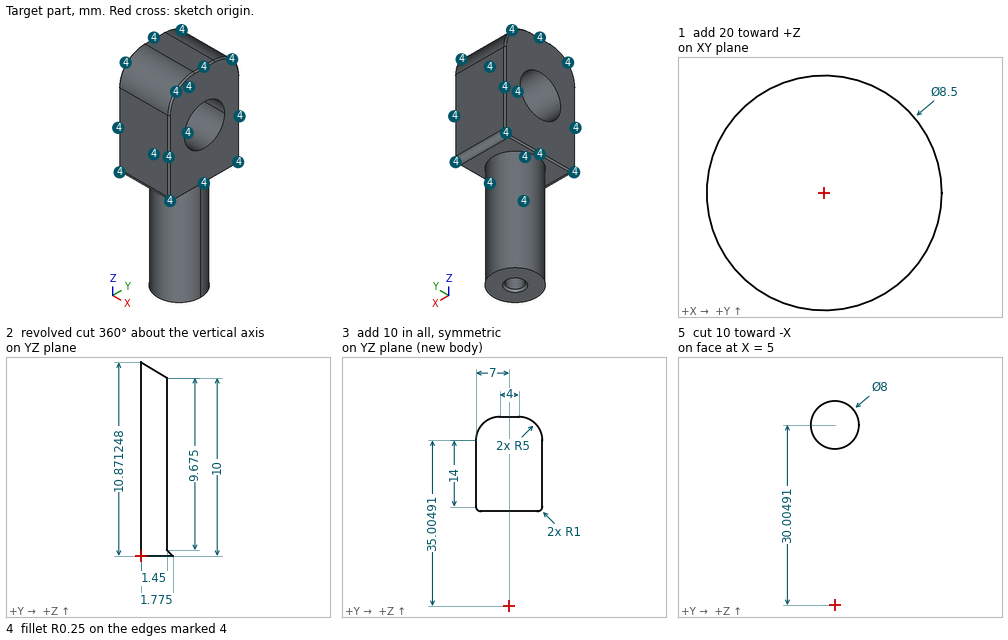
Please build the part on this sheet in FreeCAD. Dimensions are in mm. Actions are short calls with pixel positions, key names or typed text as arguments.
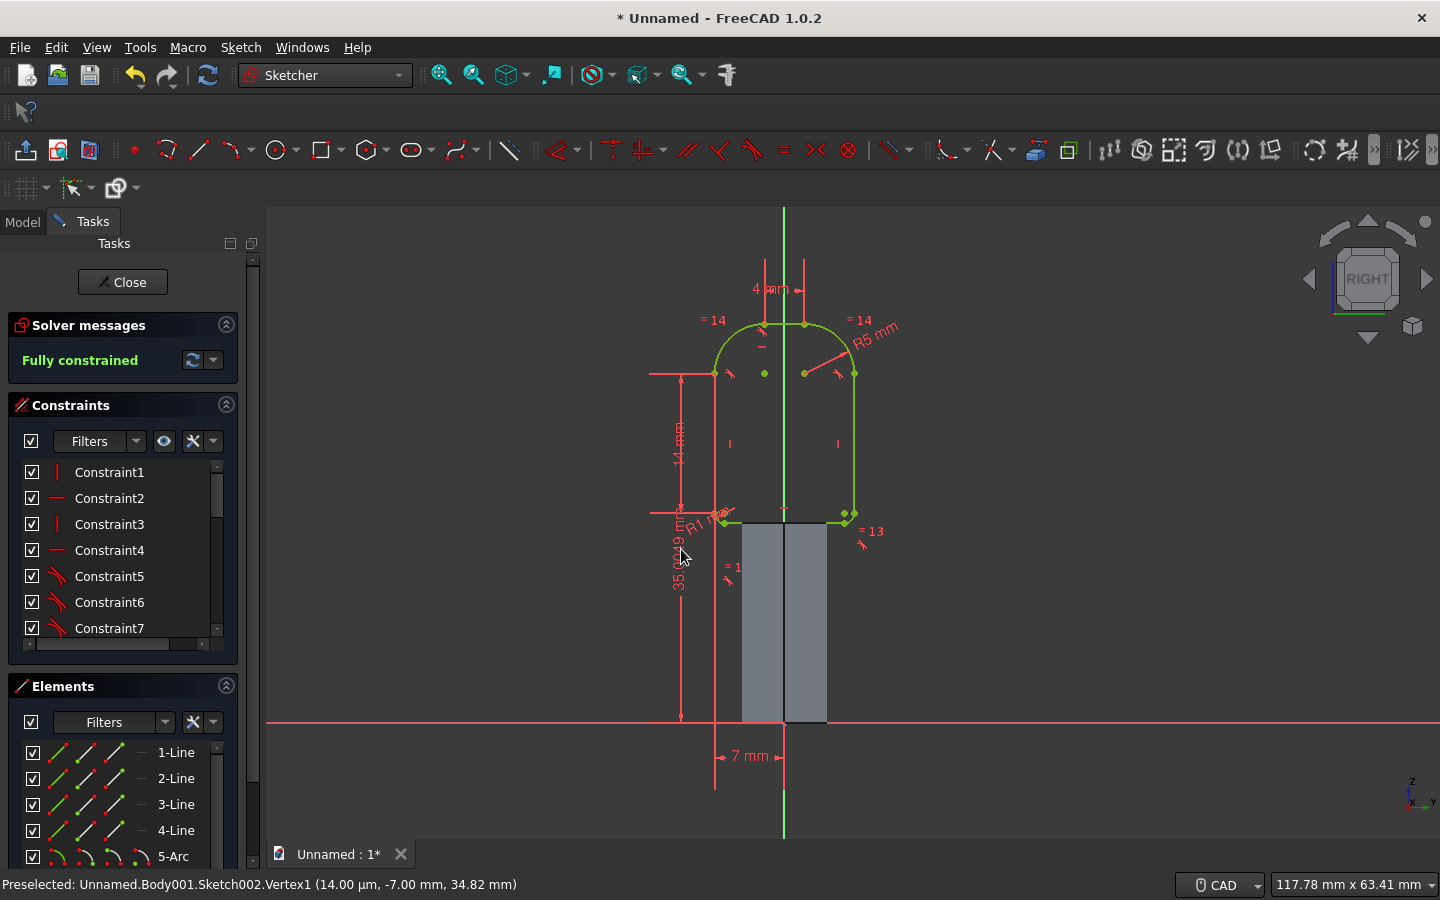
click(123, 282)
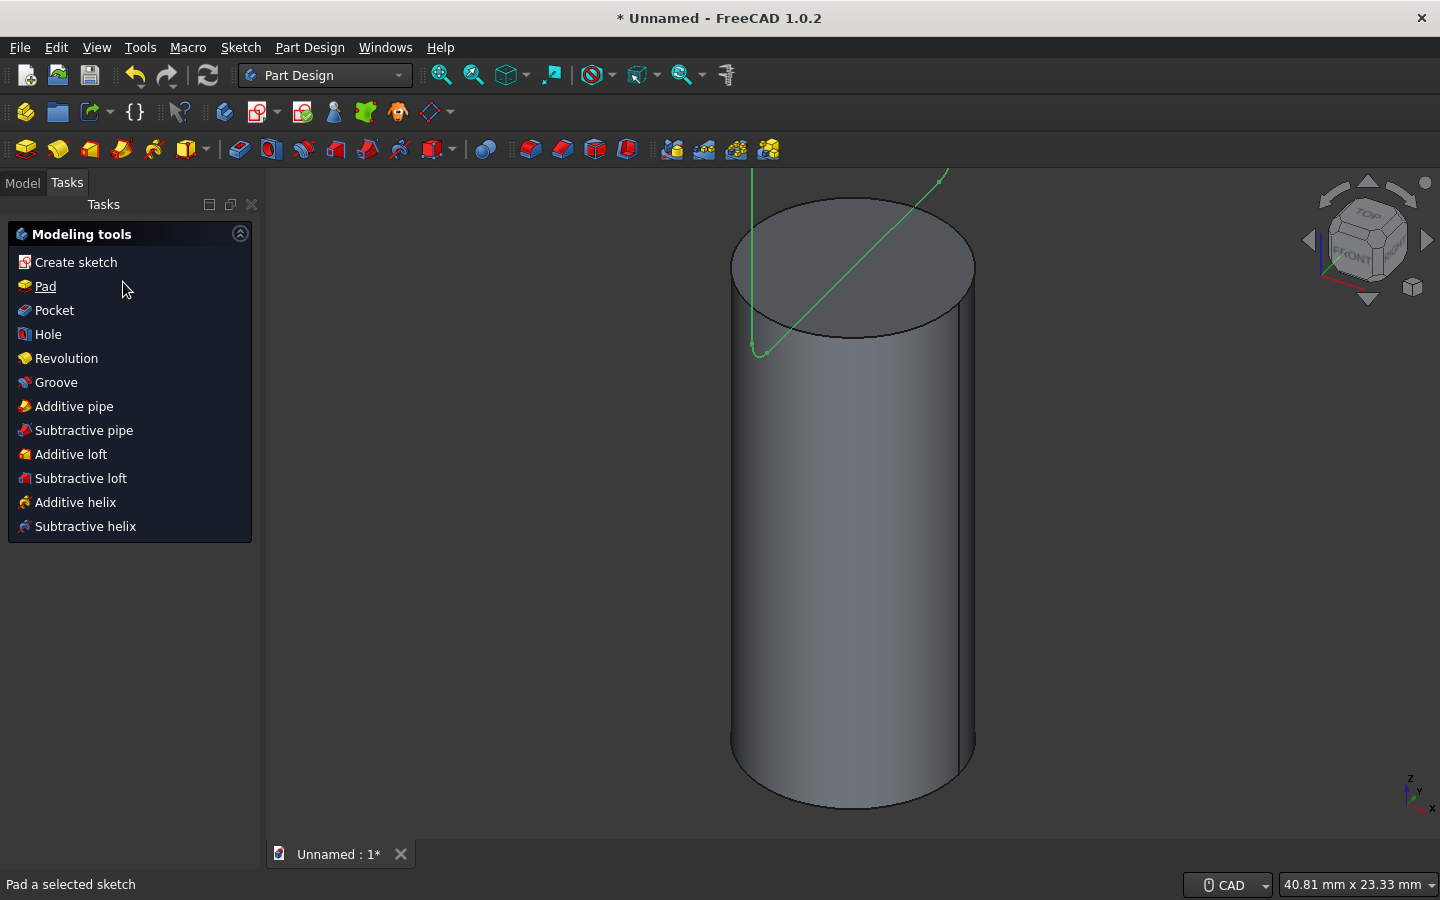
click(26, 150)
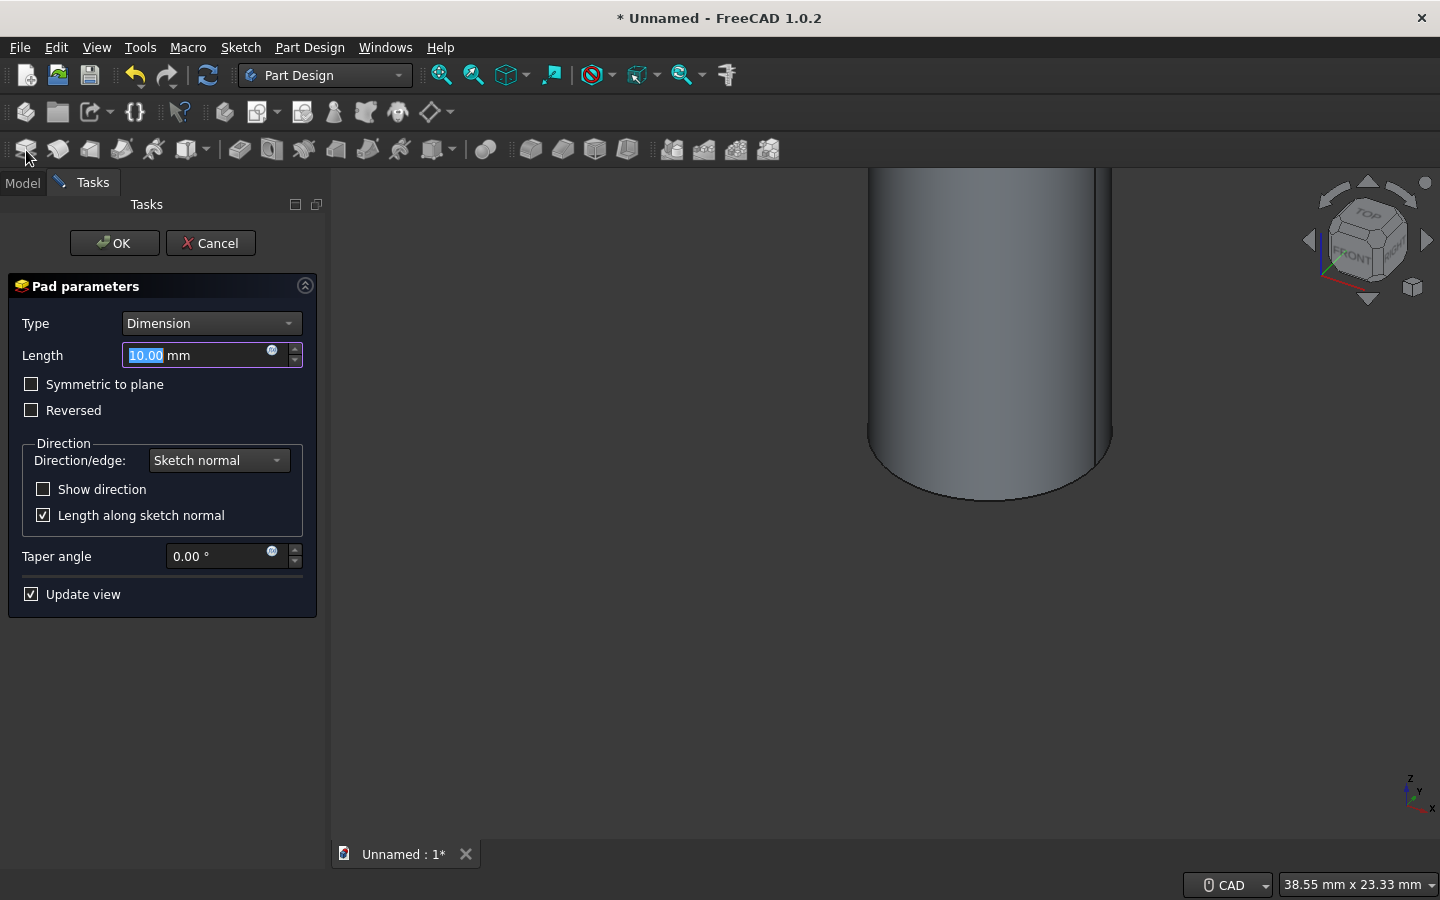
text(10)
key(Tab)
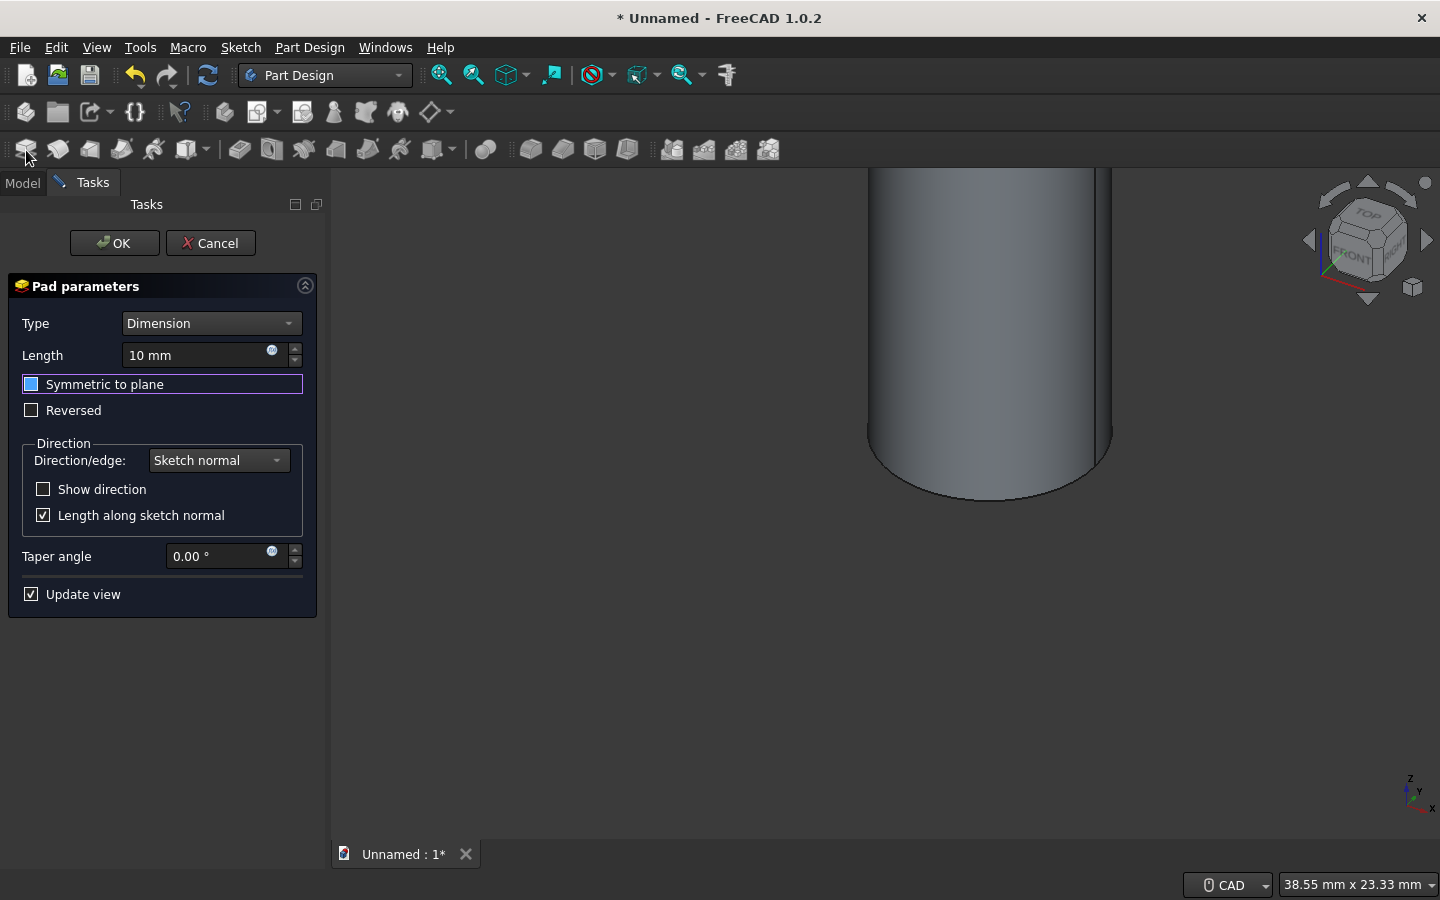
click(30, 384)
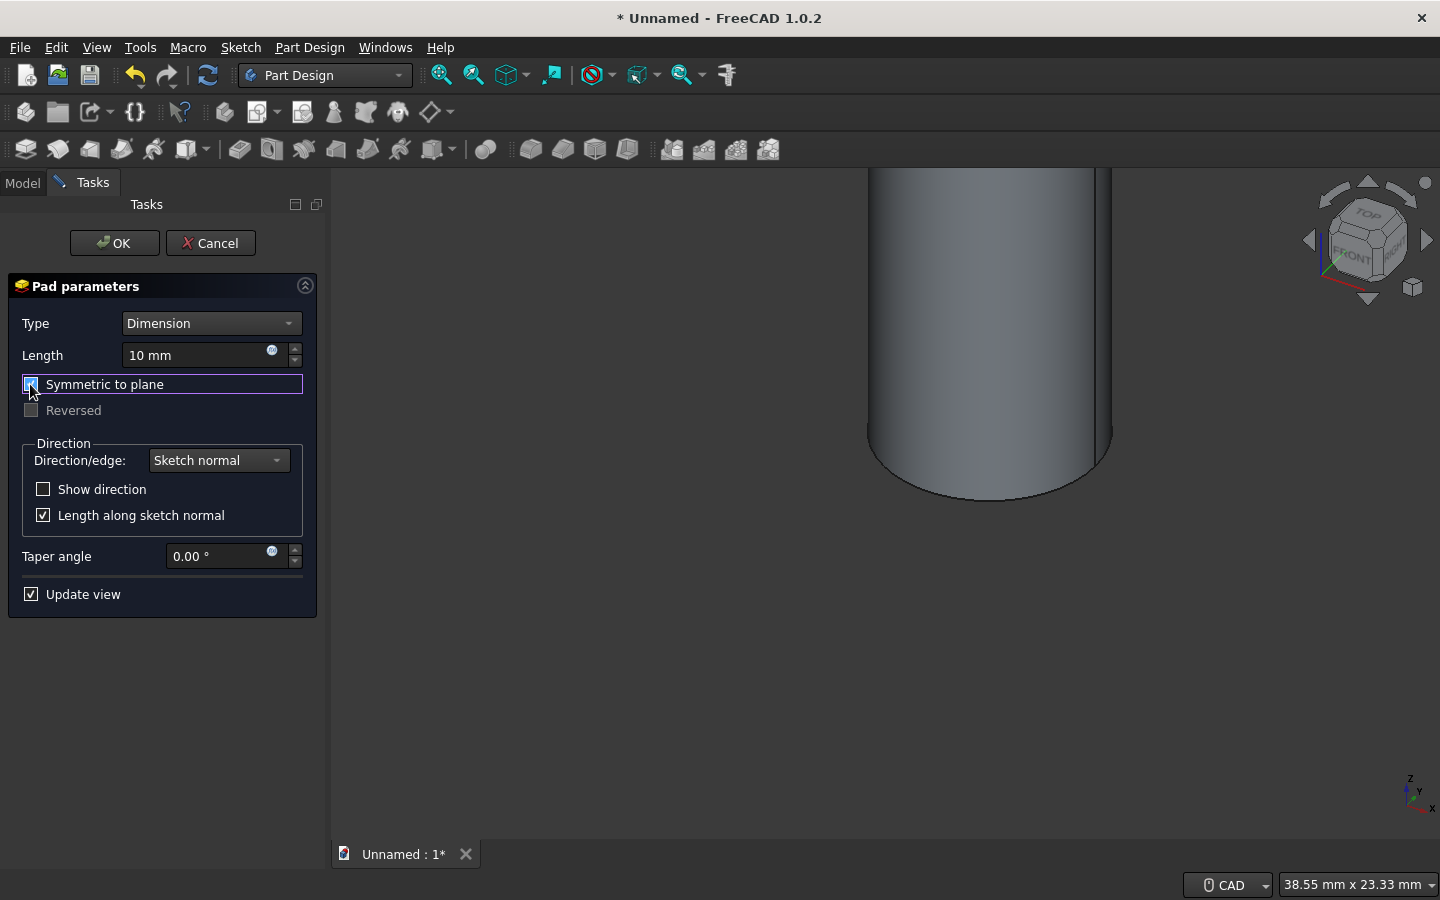
click(115, 243)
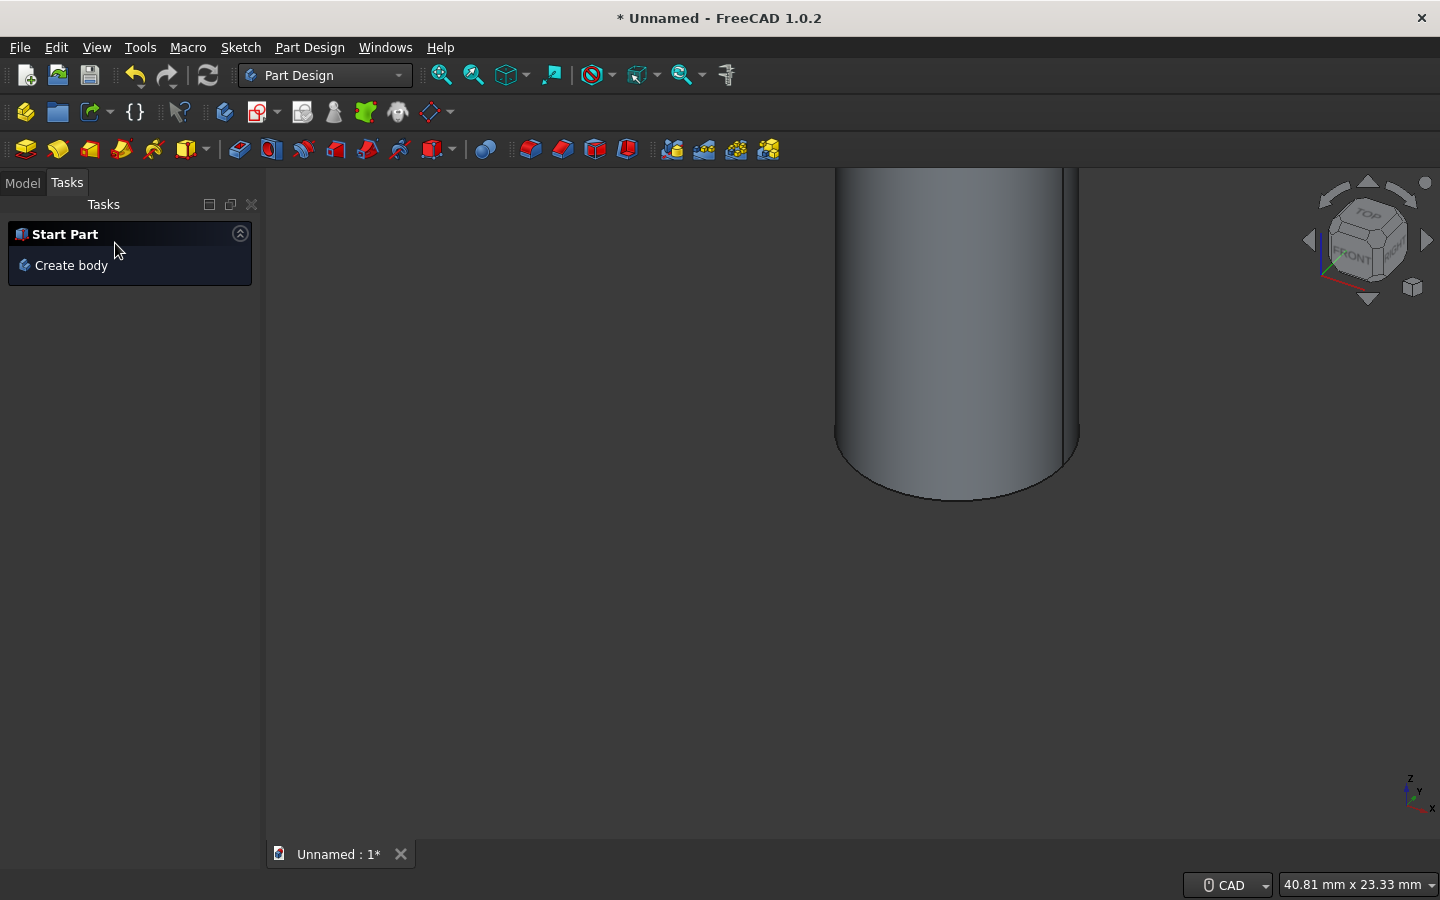
click(442, 76)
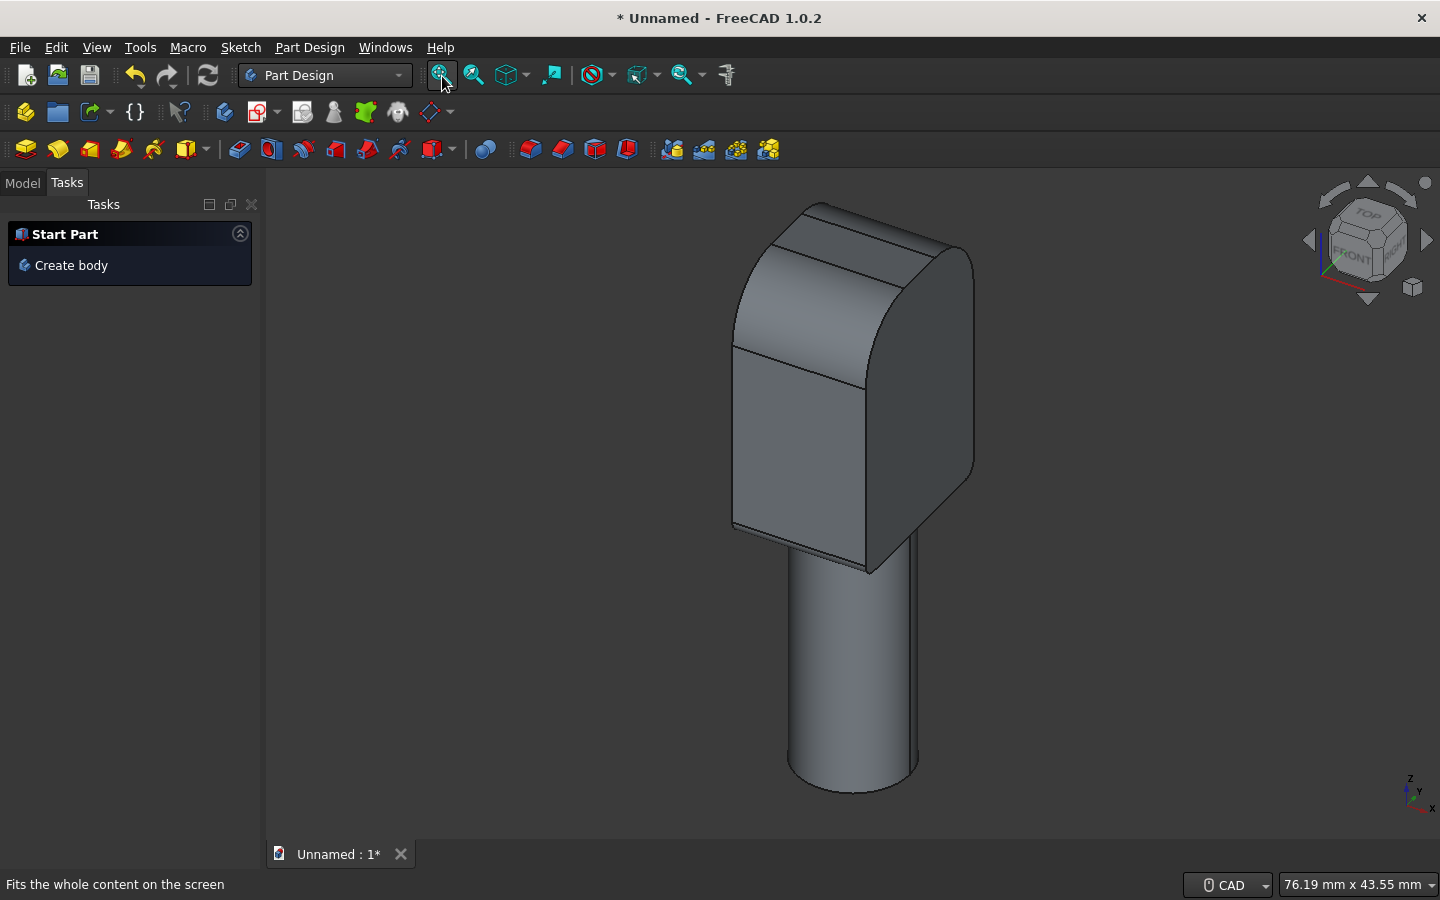
click(920, 434)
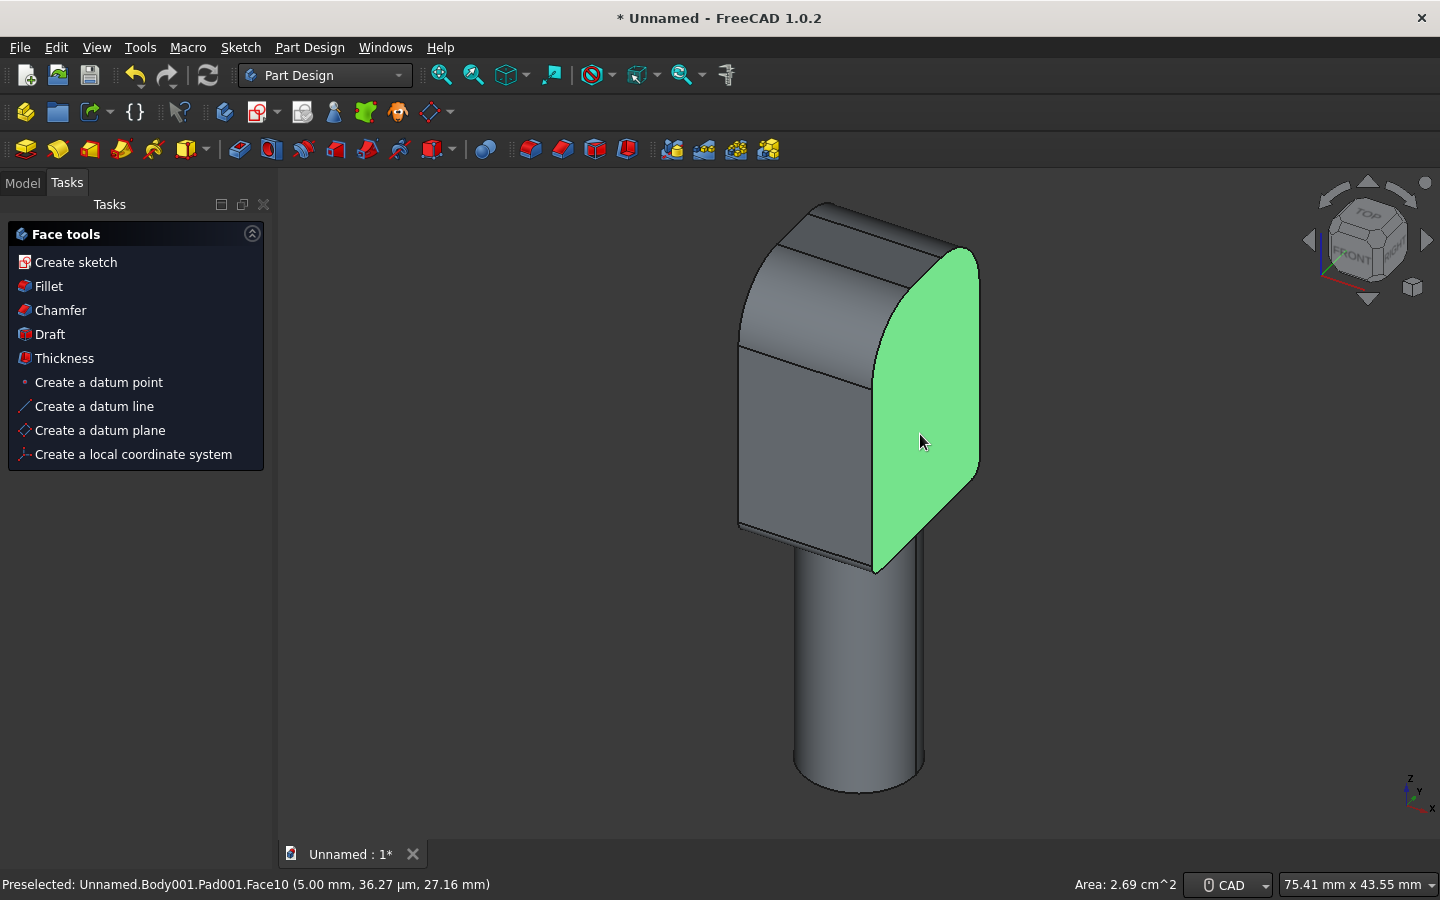
key(0)